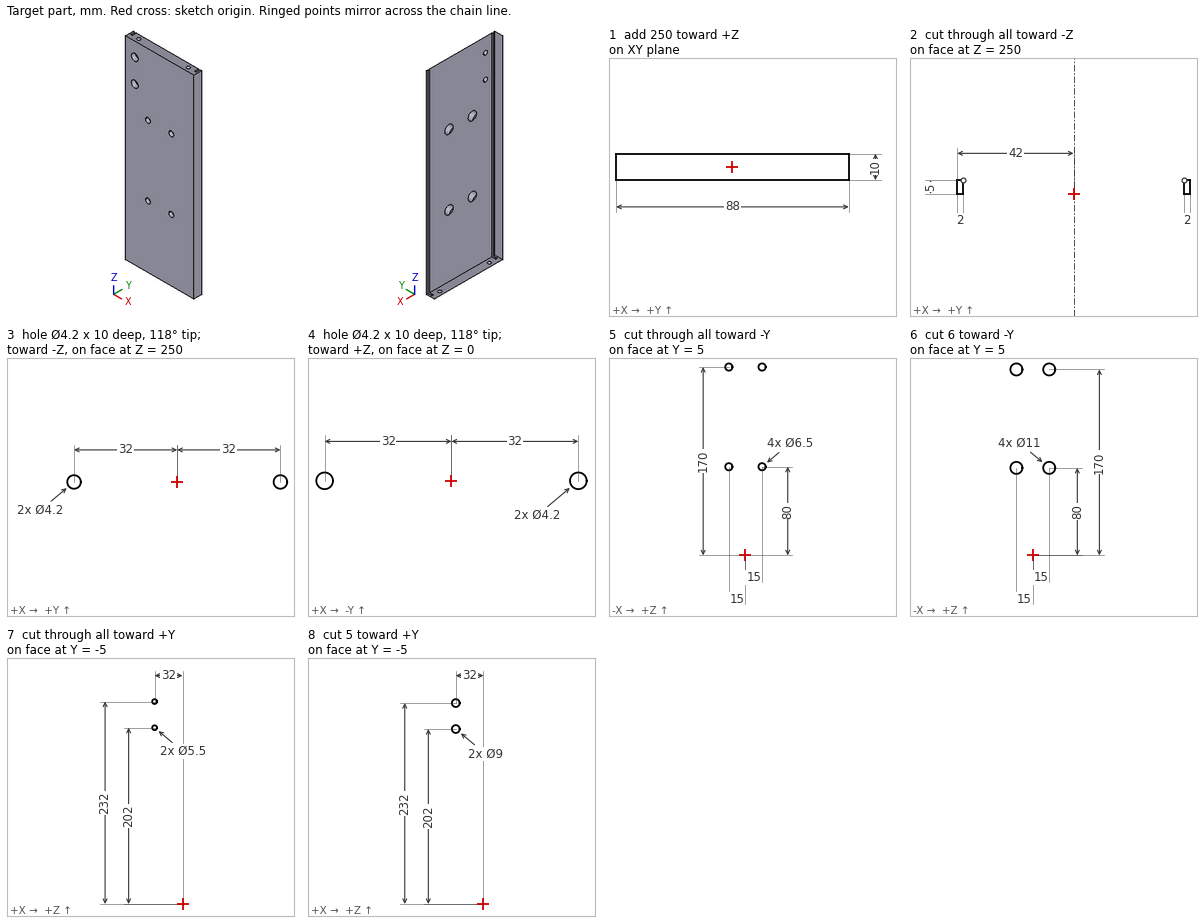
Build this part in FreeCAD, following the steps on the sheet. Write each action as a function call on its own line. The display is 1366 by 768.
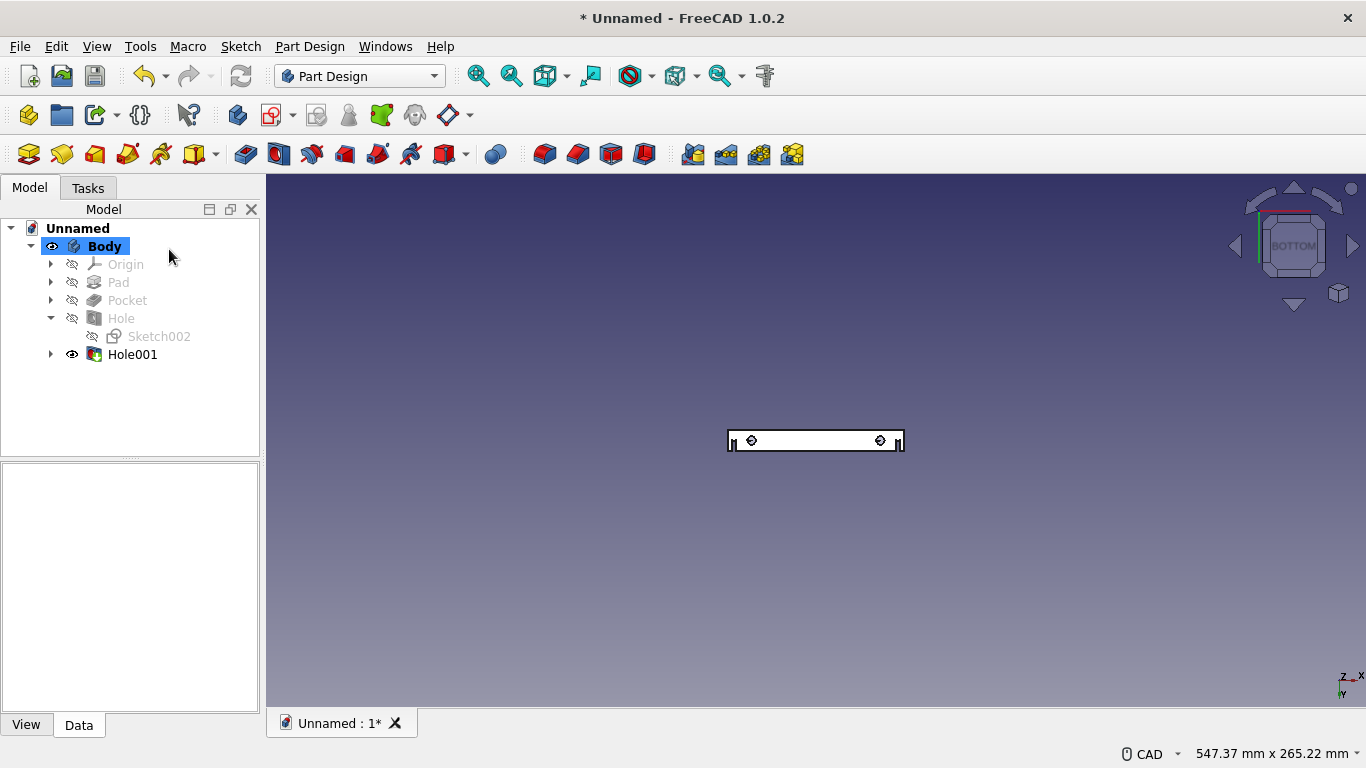
key(4)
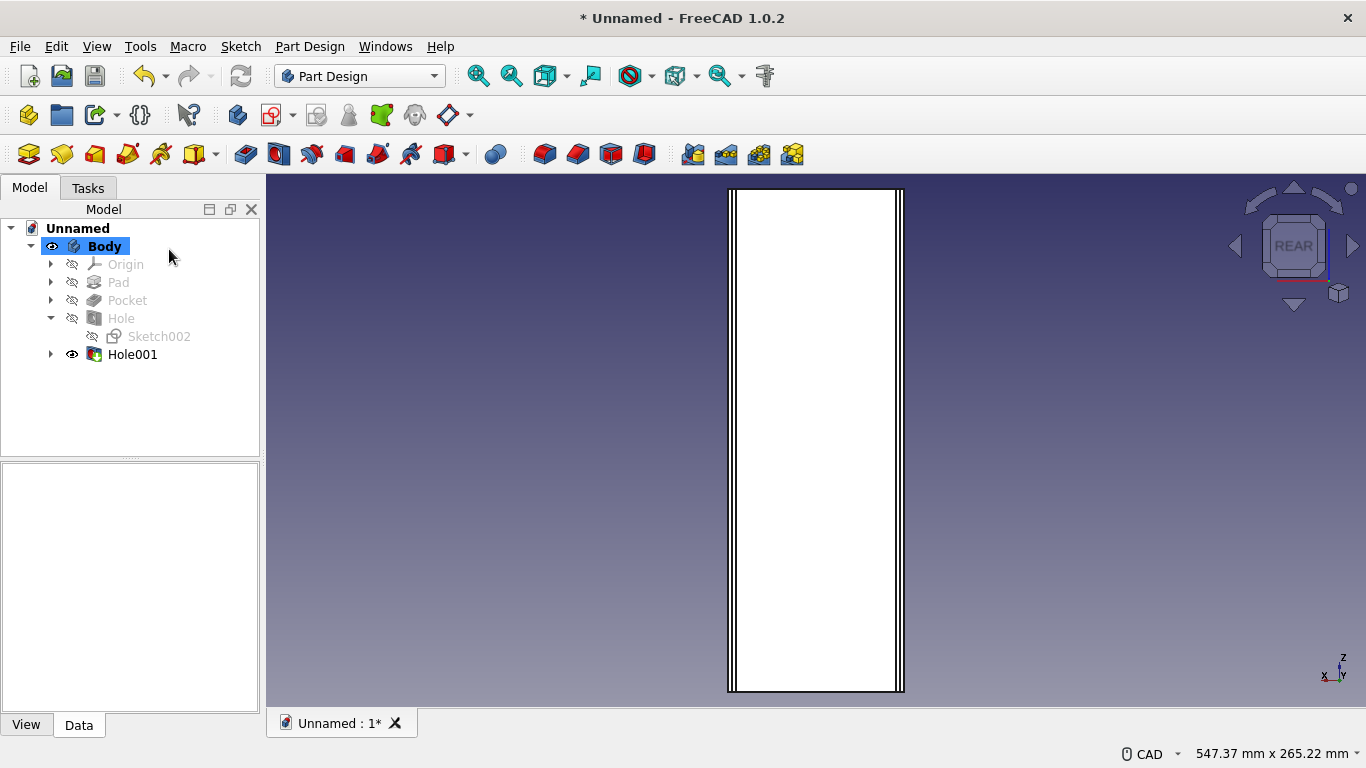
click(816, 296)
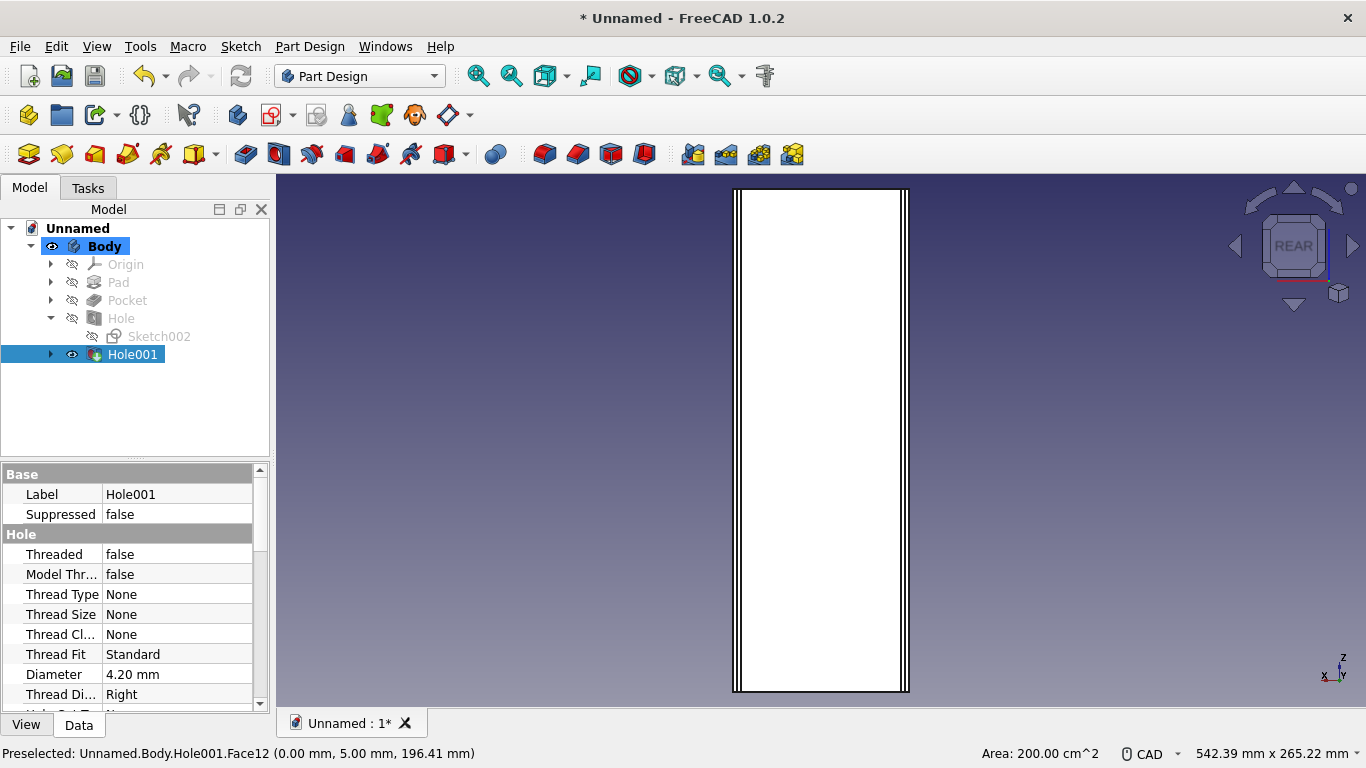
click(270, 116)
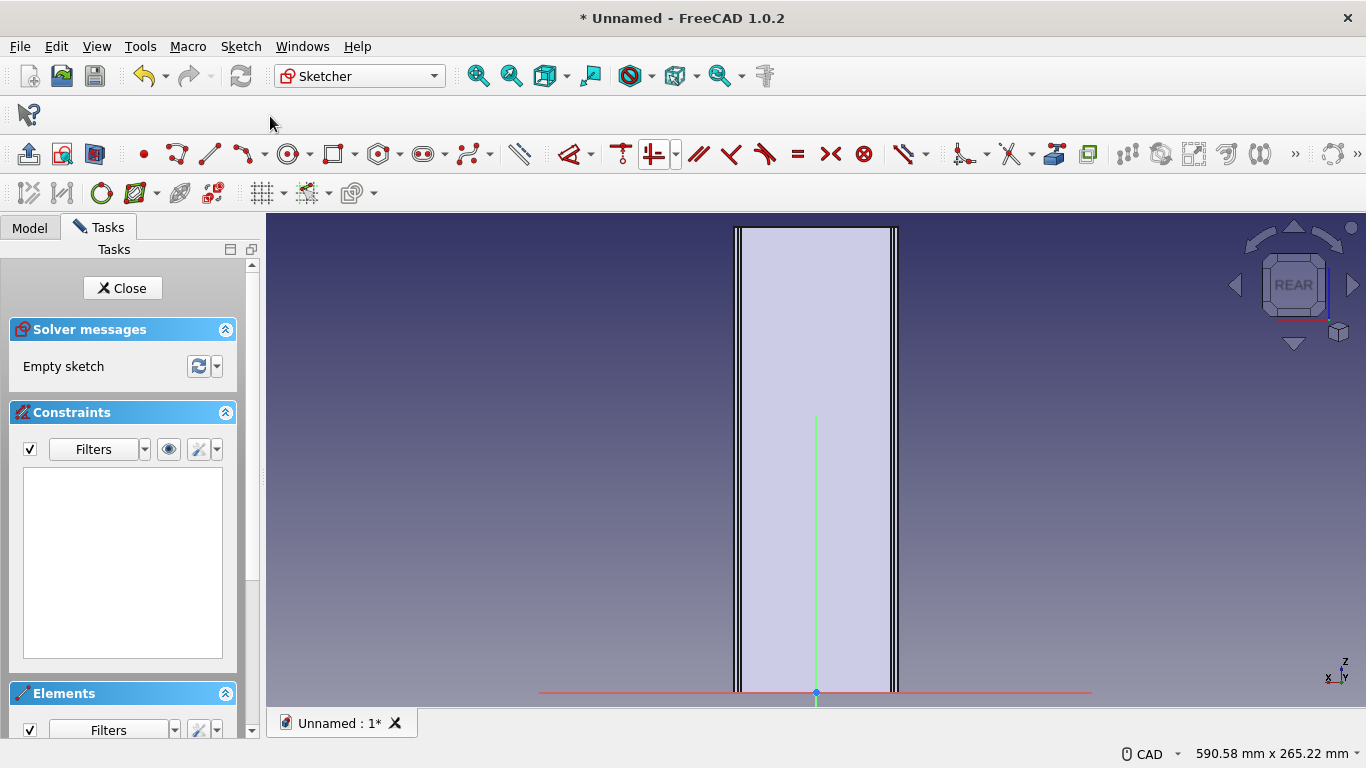
scroll(438, 241, down, 1)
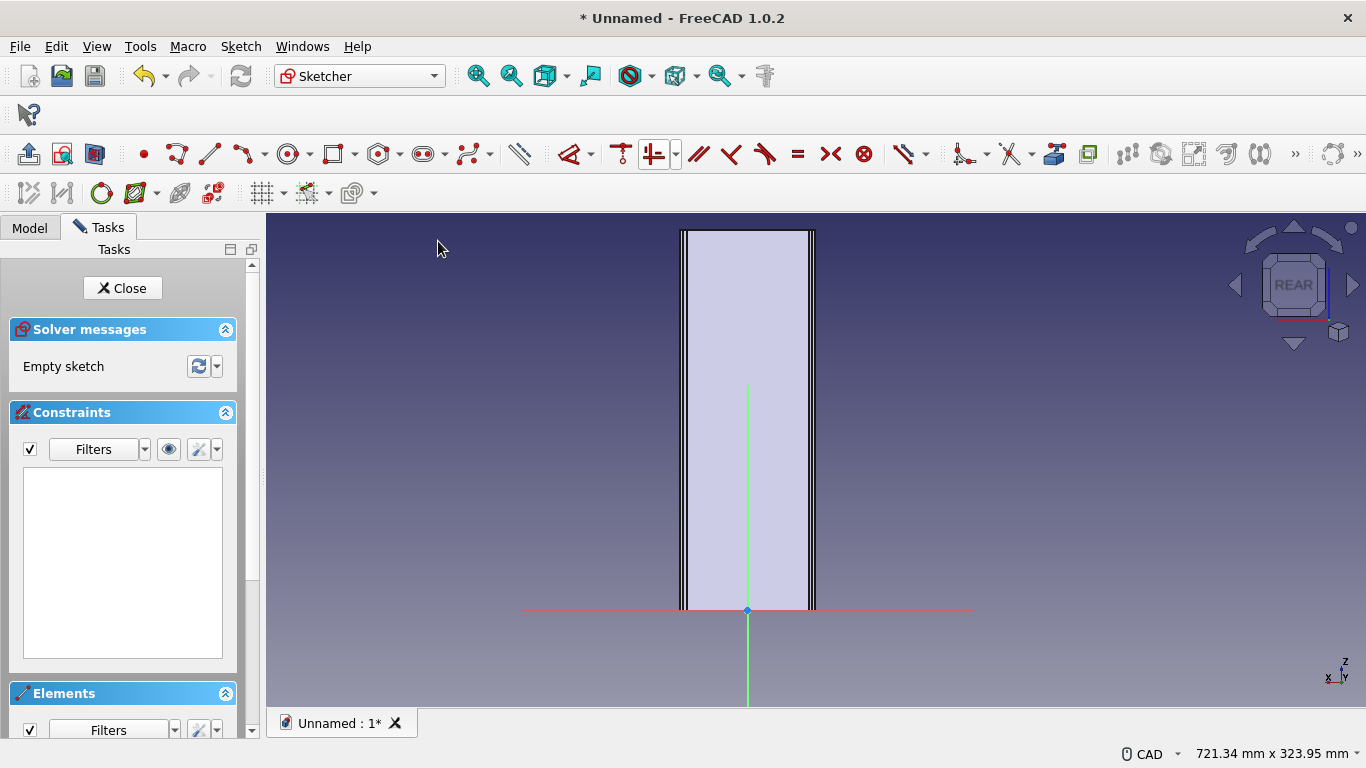
click(288, 154)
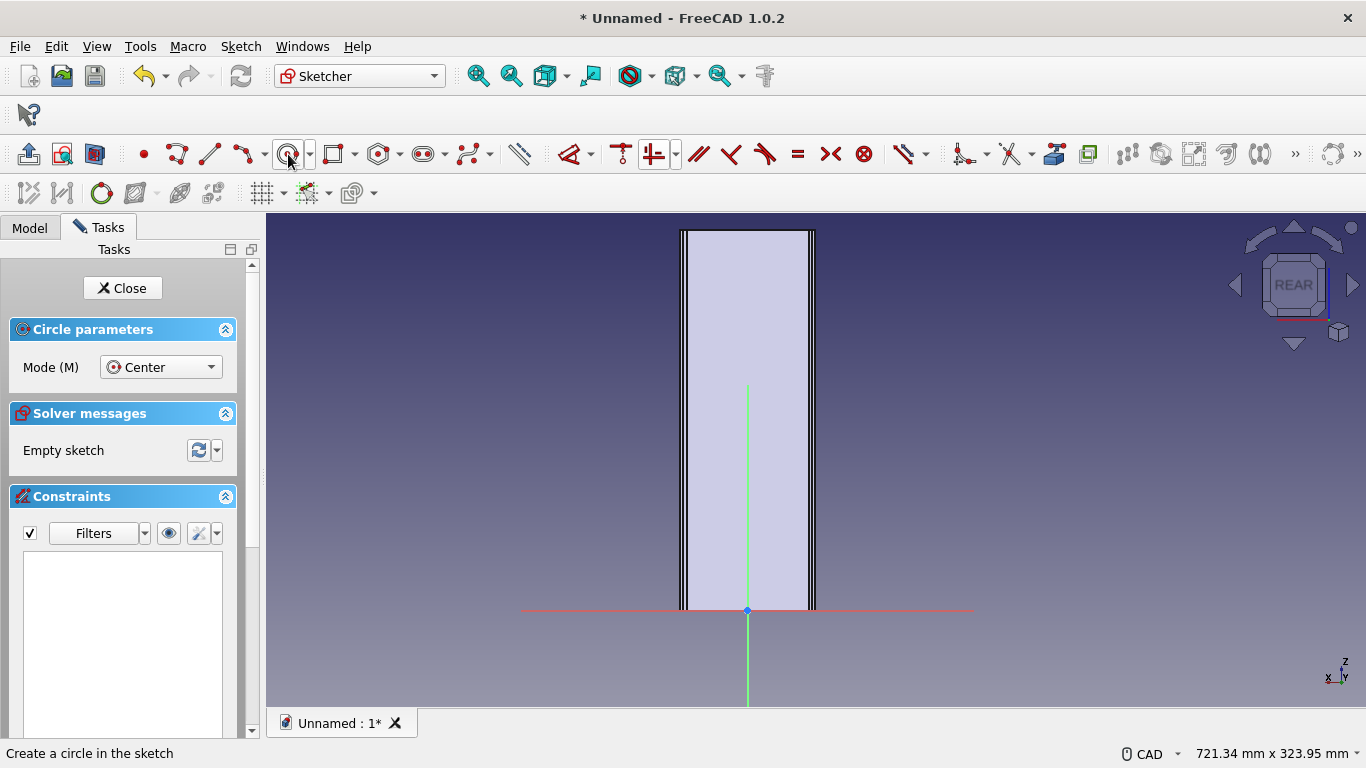
scroll(770, 489, up, 8)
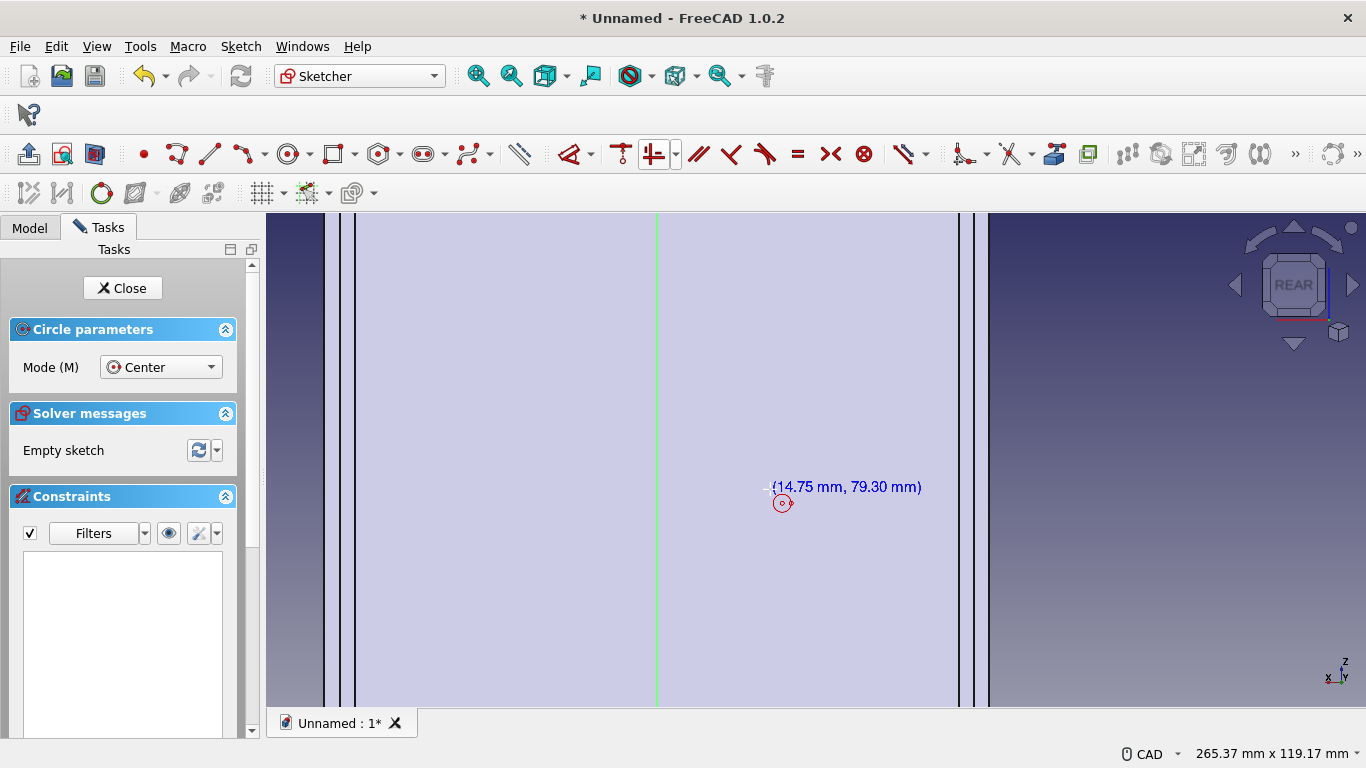
scroll(777, 468, down, 7)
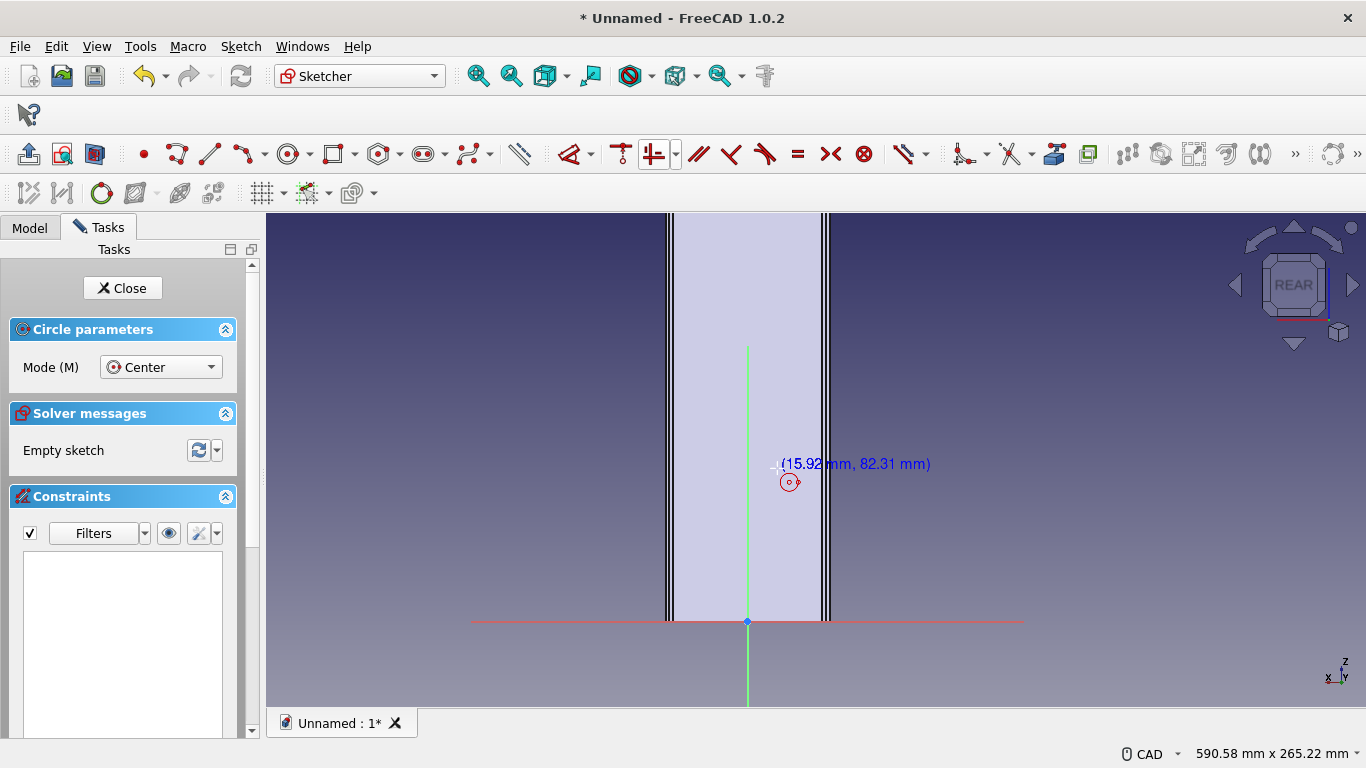
click(776, 473)
move(780, 469)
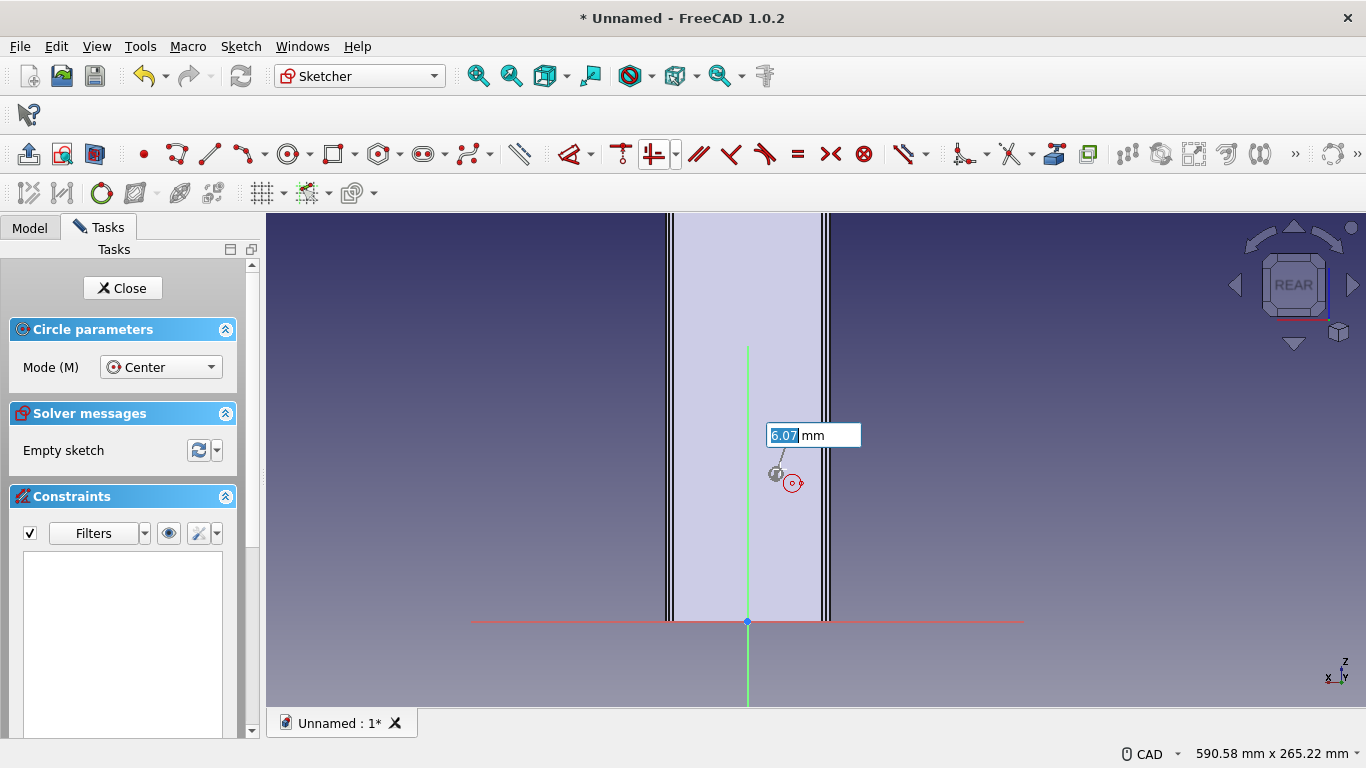
text(6.5)
key(Return)